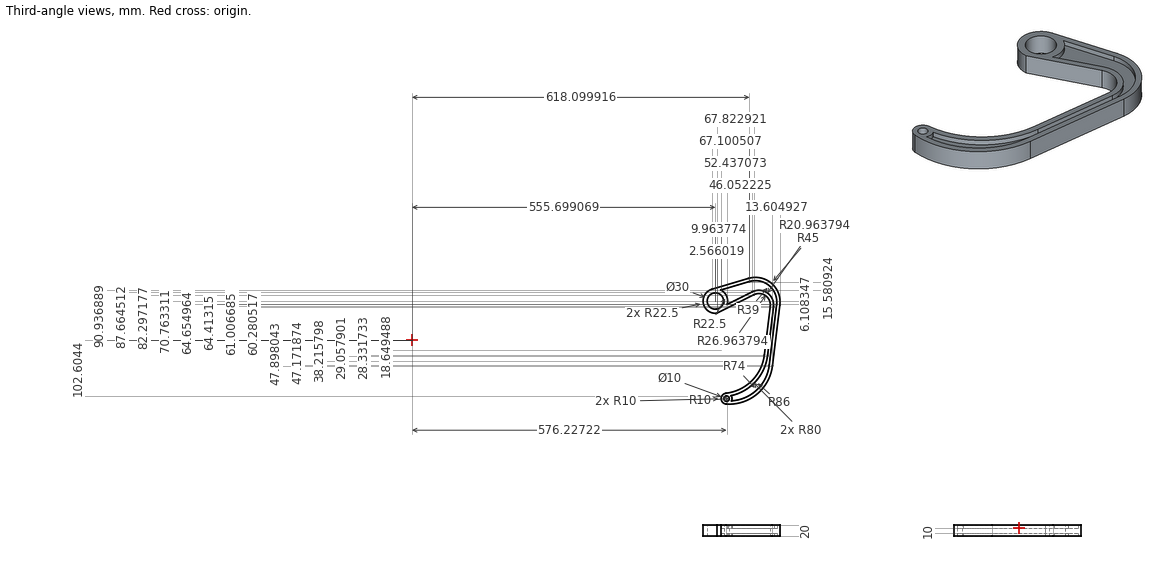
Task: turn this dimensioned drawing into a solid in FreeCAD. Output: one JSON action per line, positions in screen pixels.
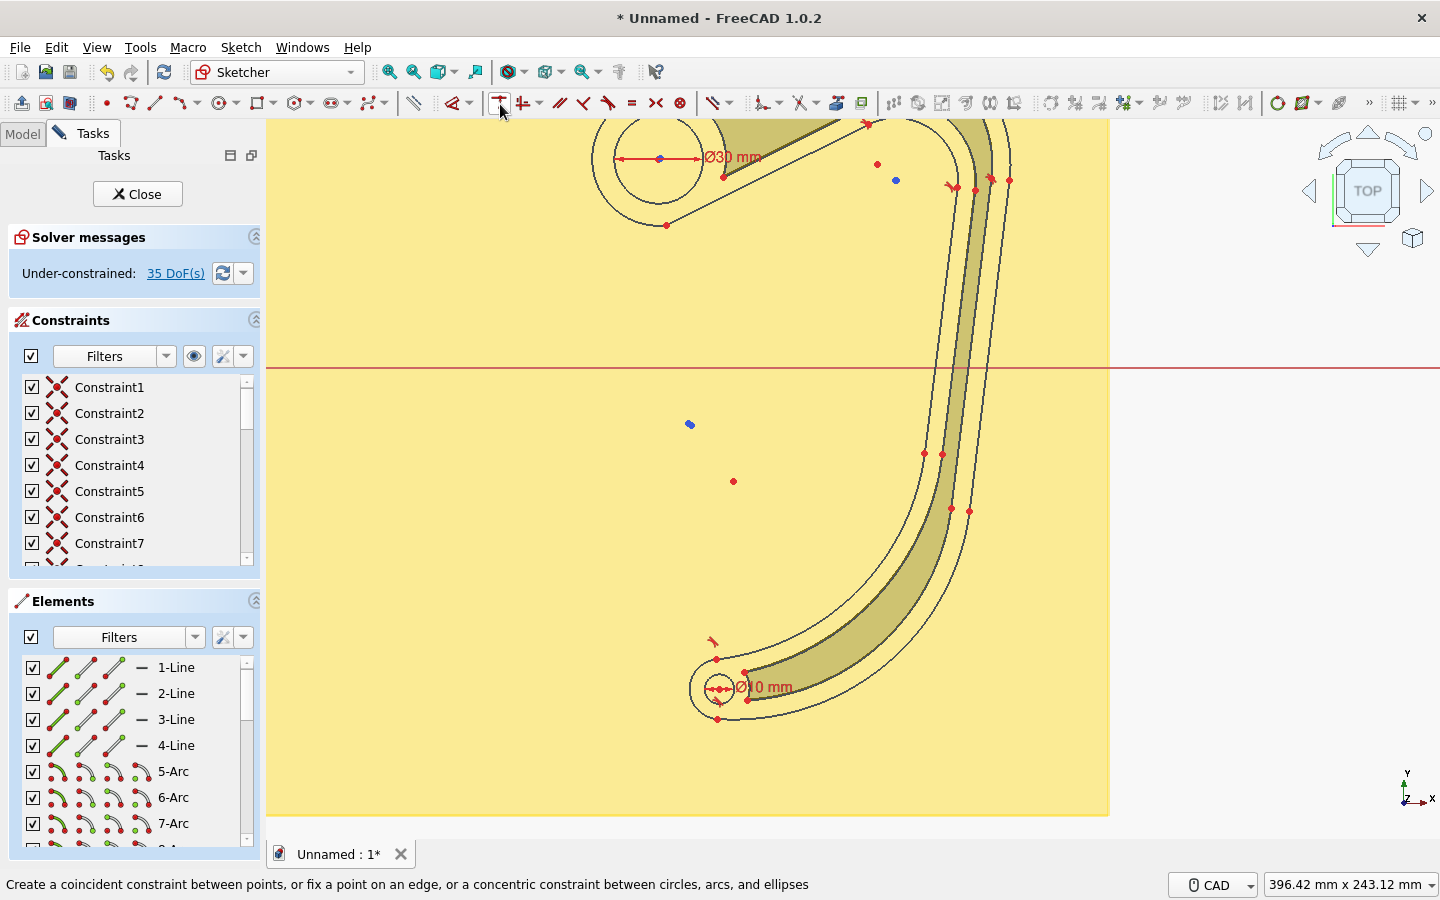
{"action": "left_click", "coordinate": [806, 630]}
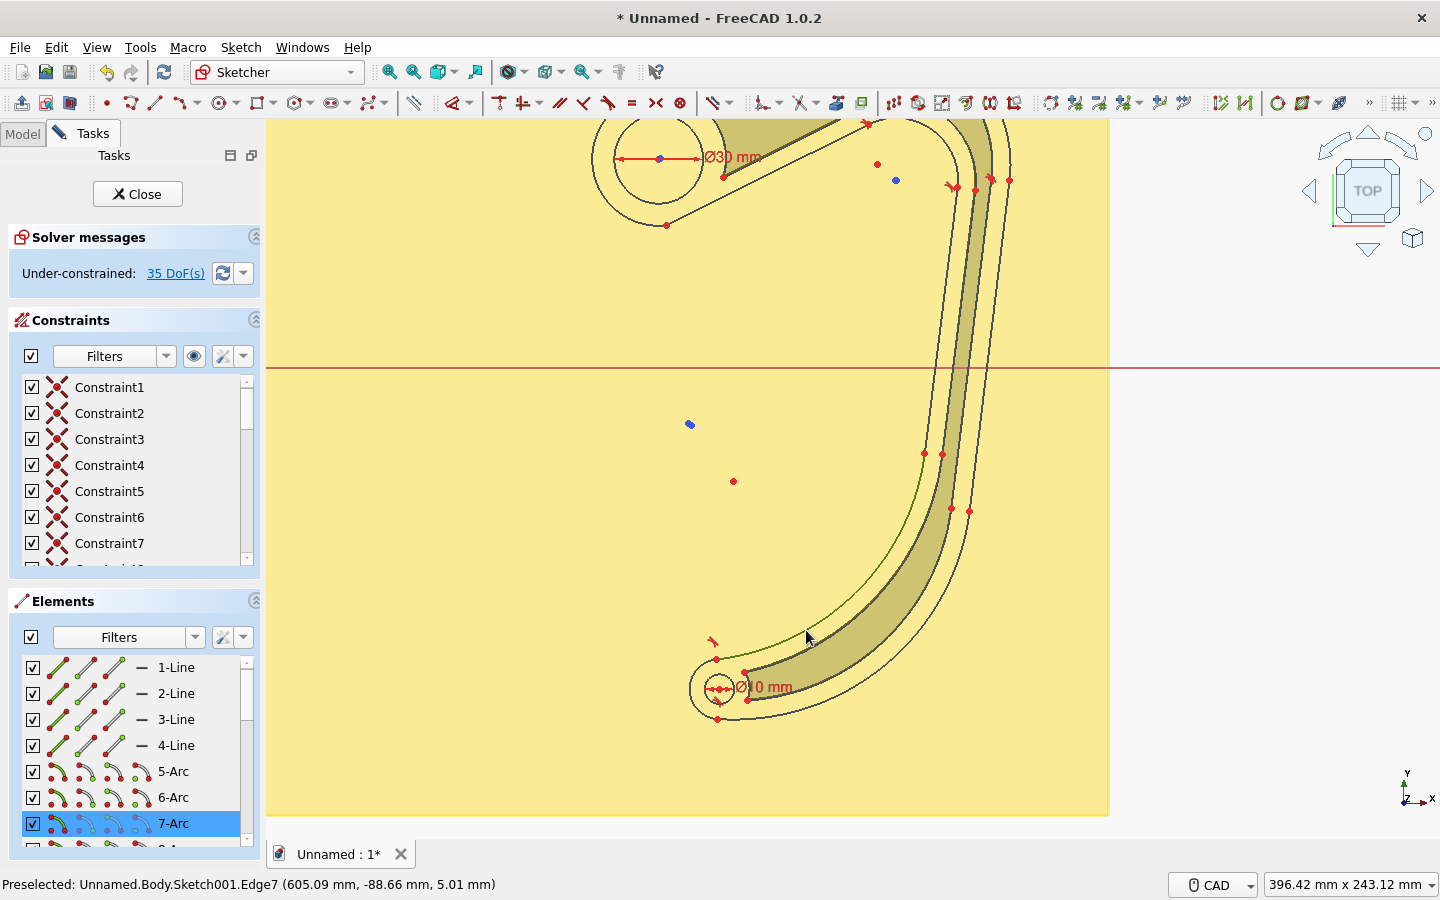
{"action": "left_click", "coordinate": [831, 636]}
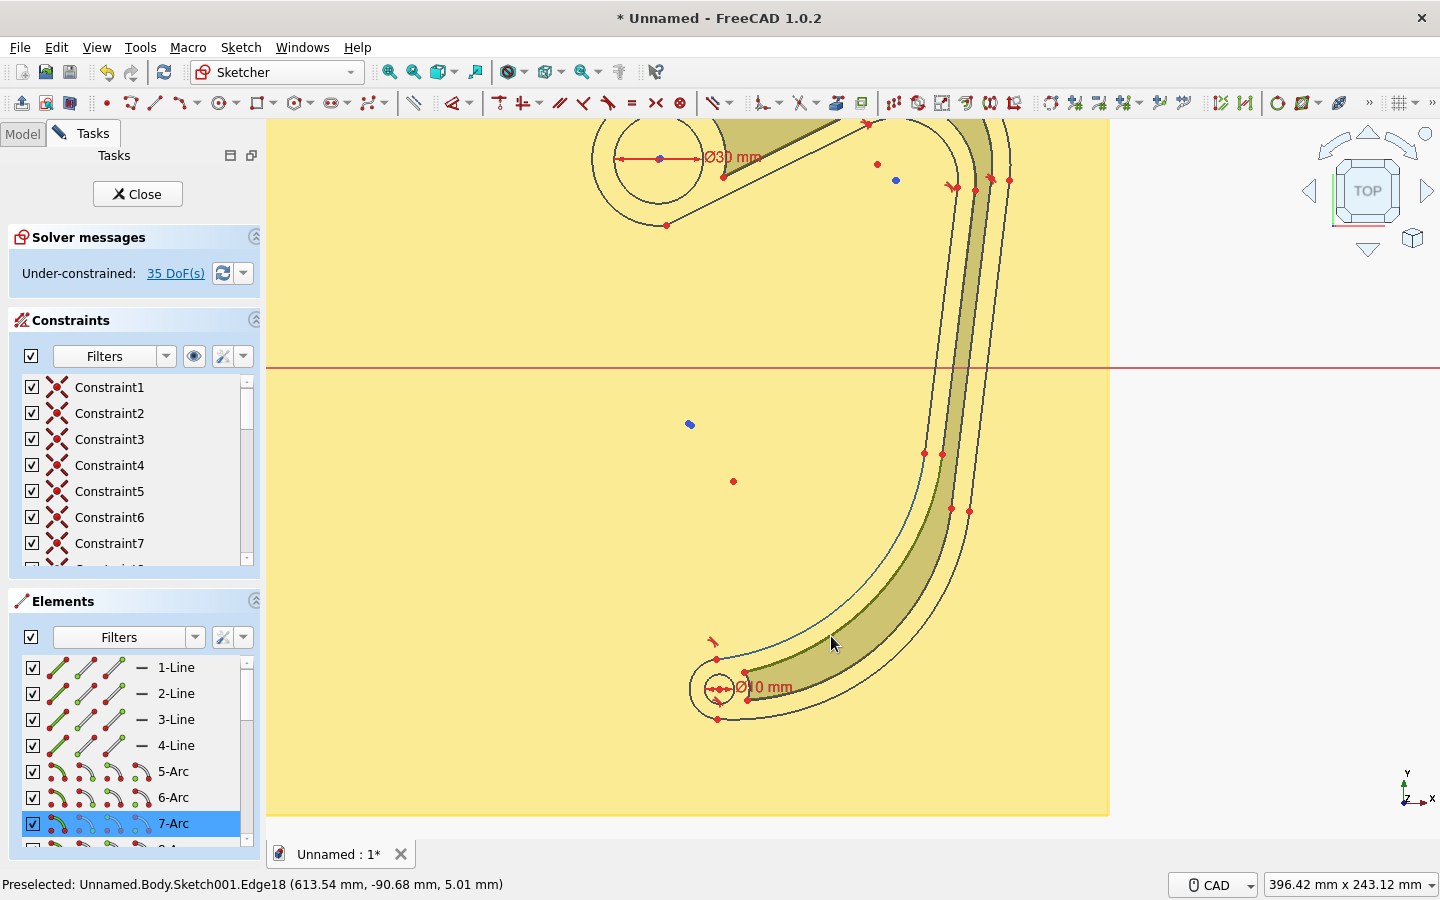
{"action": "key", "text": "c"}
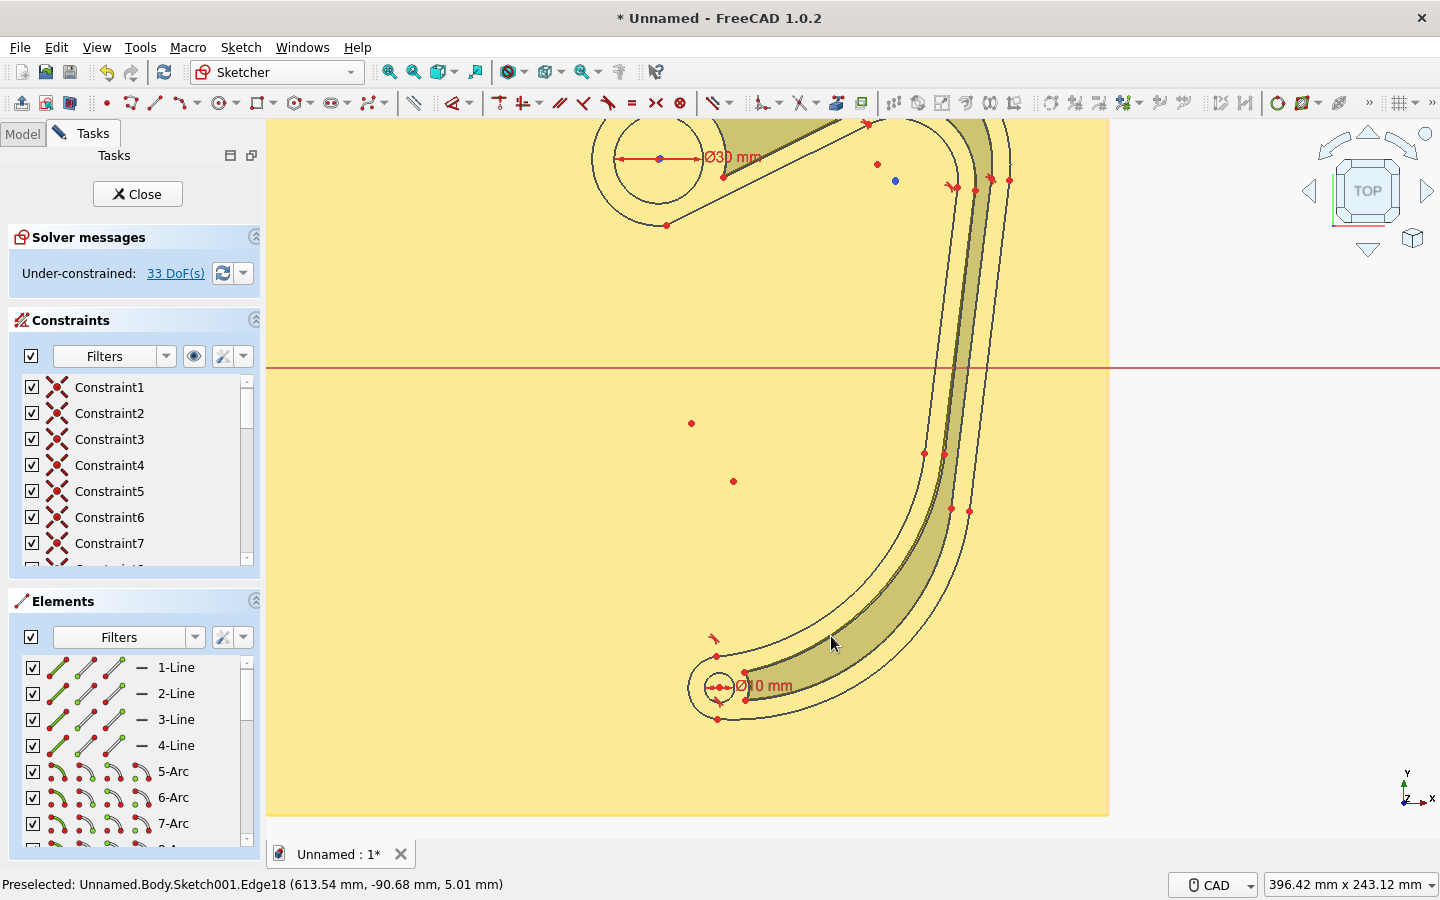
{"action": "left_click", "coordinate": [950, 149]}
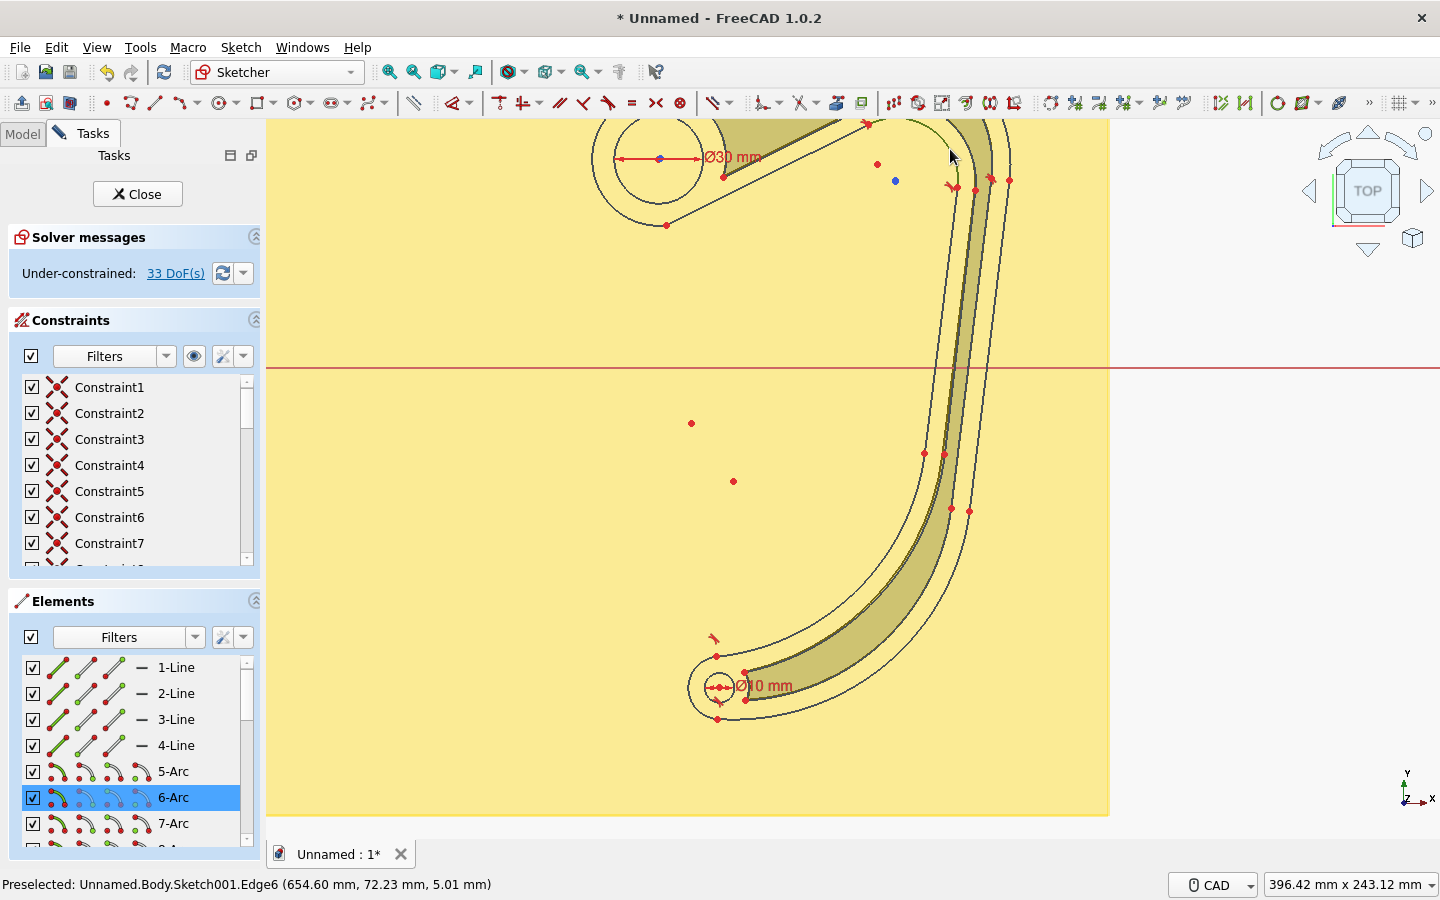
{"action": "left_click", "coordinate": [972, 157]}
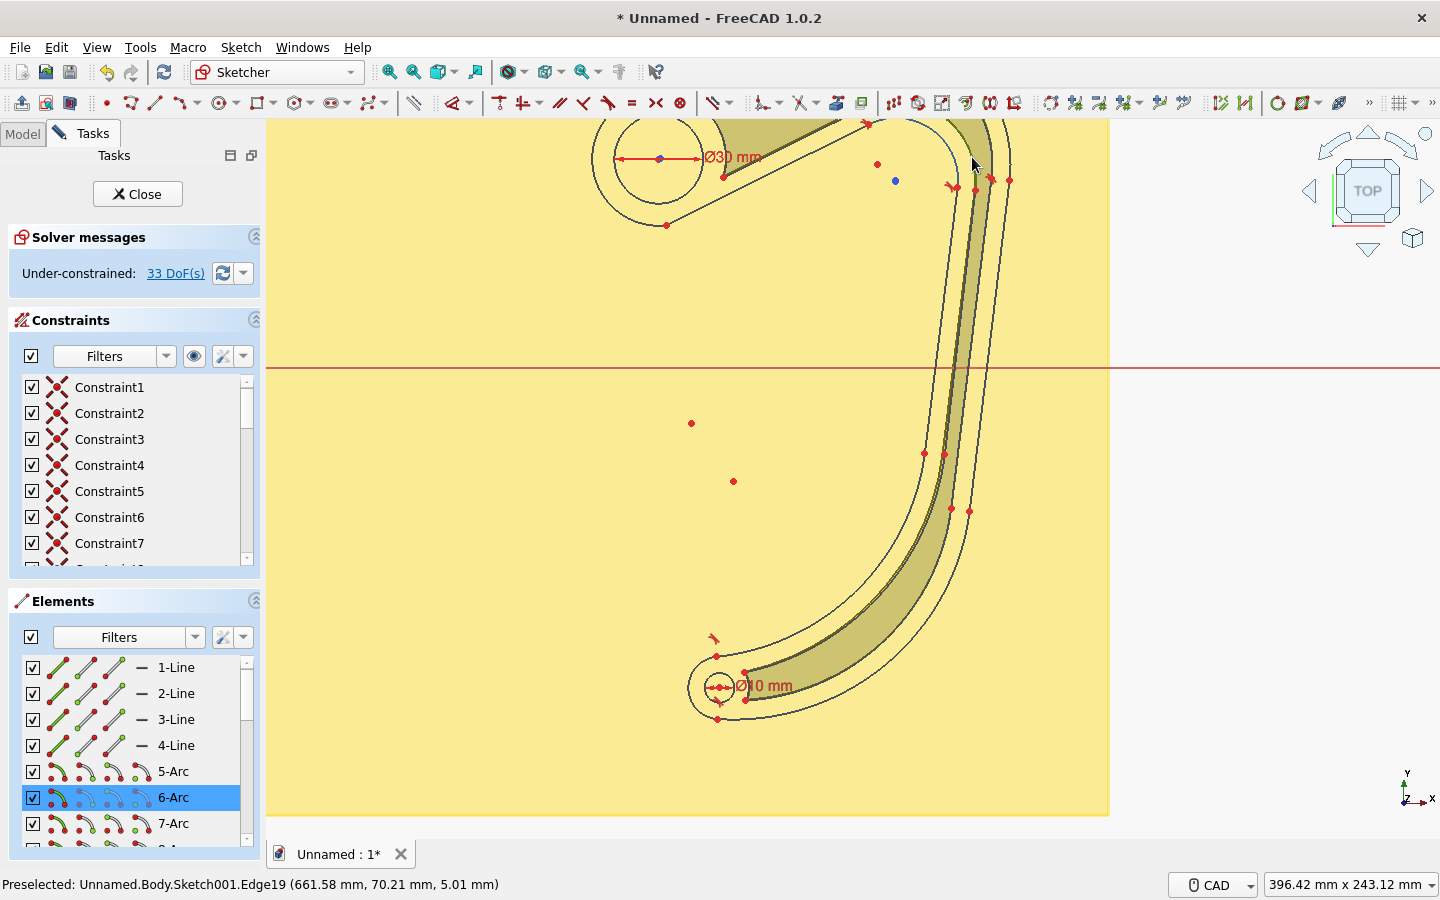
{"action": "left_click", "coordinate": [500, 104]}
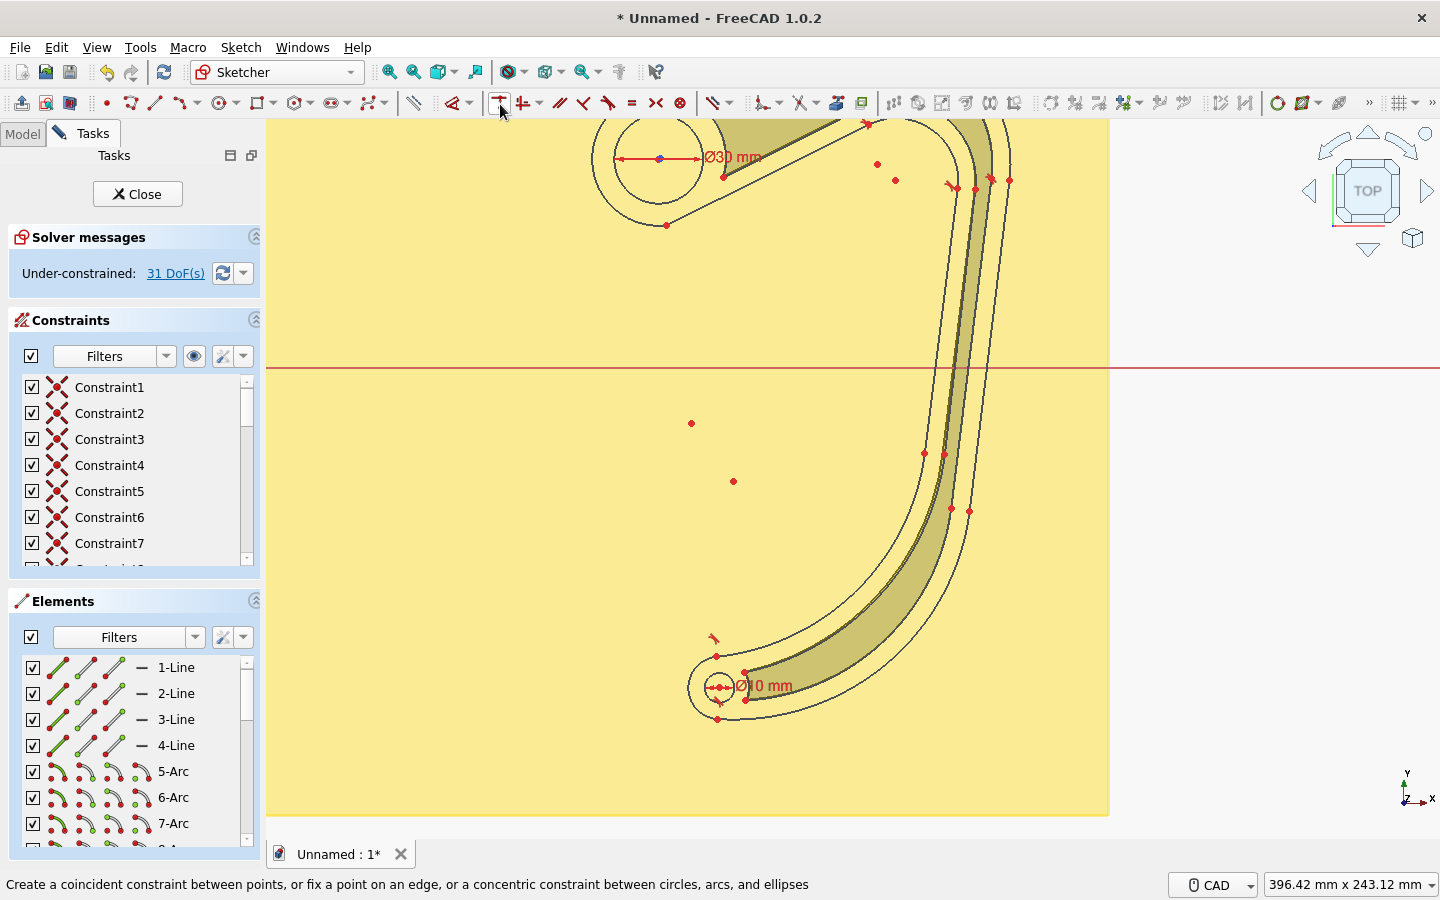
{"action": "left_click", "coordinate": [627, 191]}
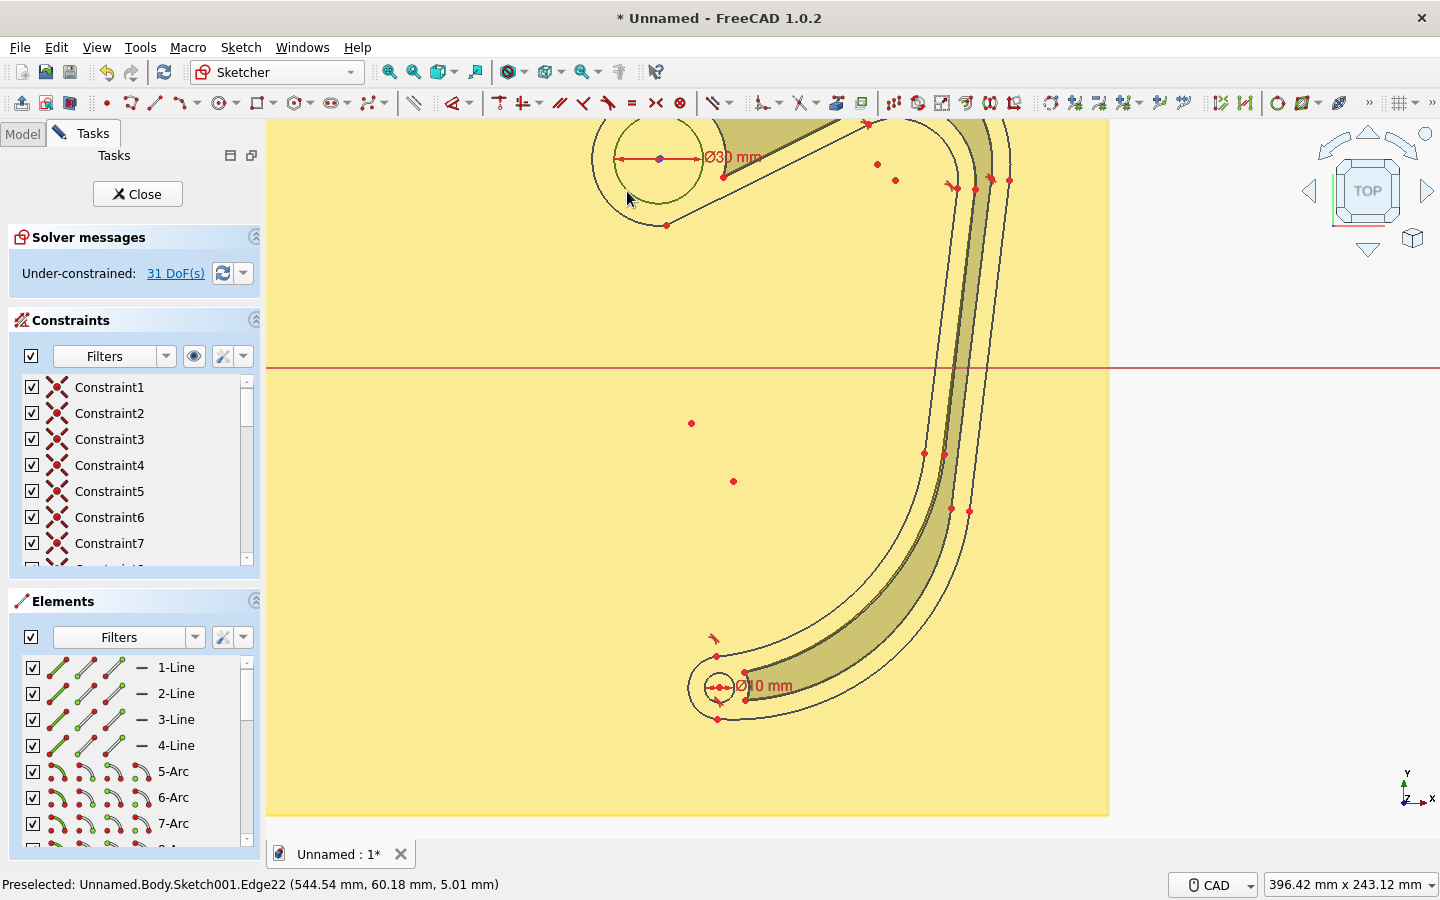
{"action": "left_click", "coordinate": [726, 150]}